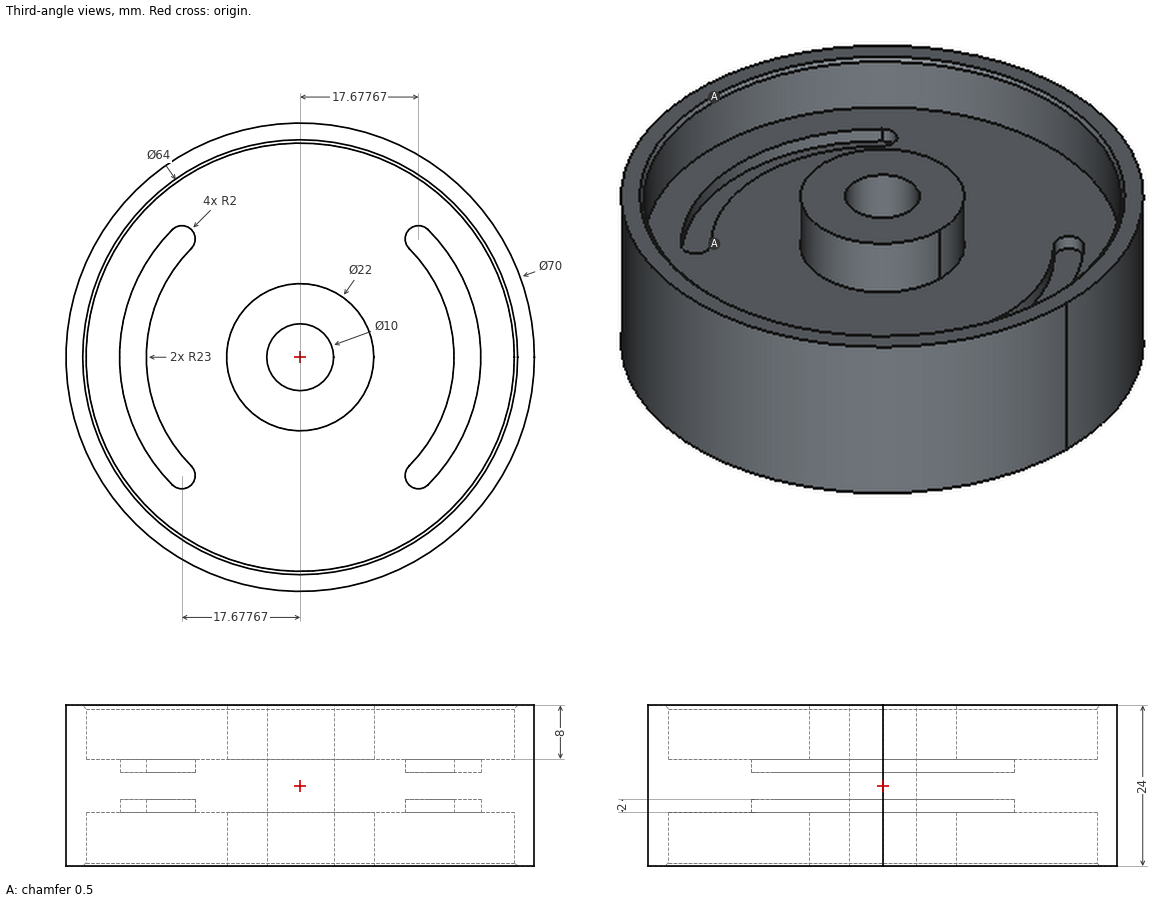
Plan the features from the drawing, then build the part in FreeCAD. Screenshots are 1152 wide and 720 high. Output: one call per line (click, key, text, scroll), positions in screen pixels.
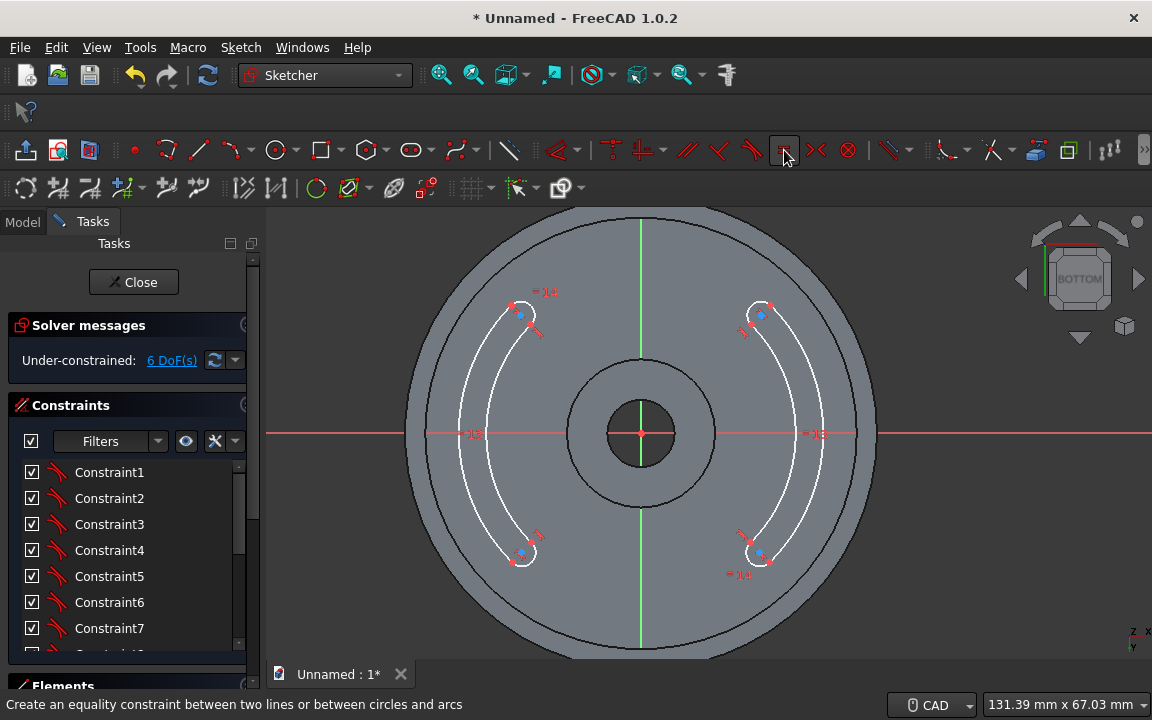
key(d)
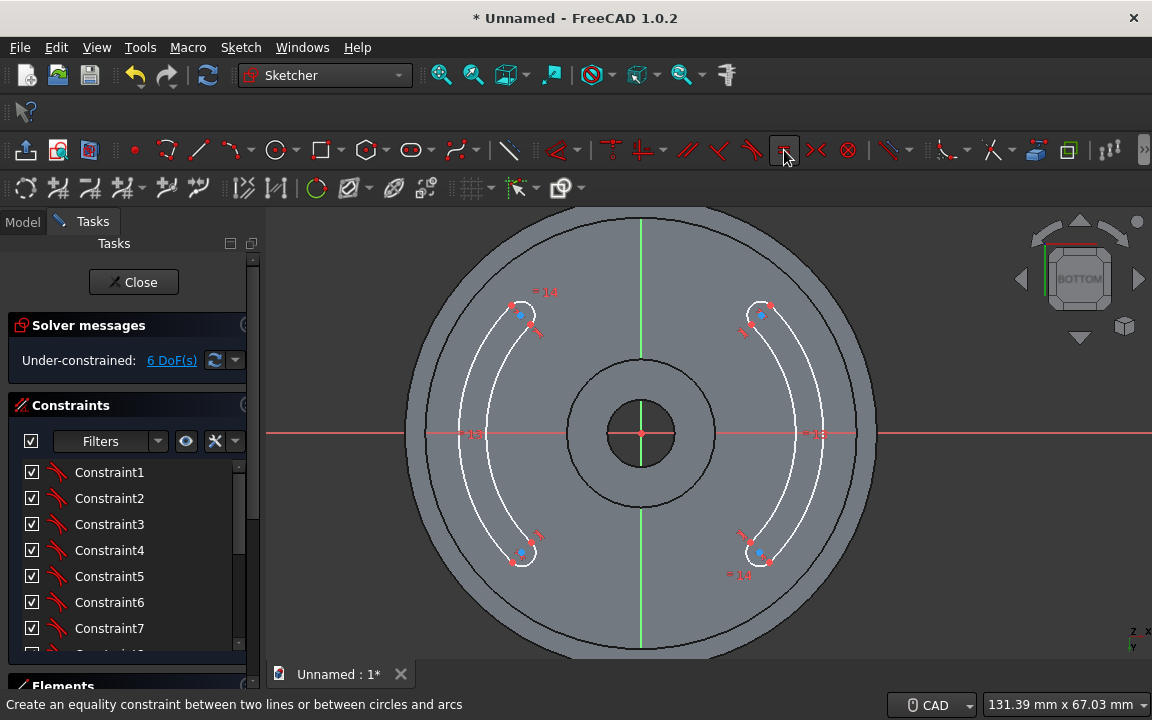
click(494, 387)
click(592, 254)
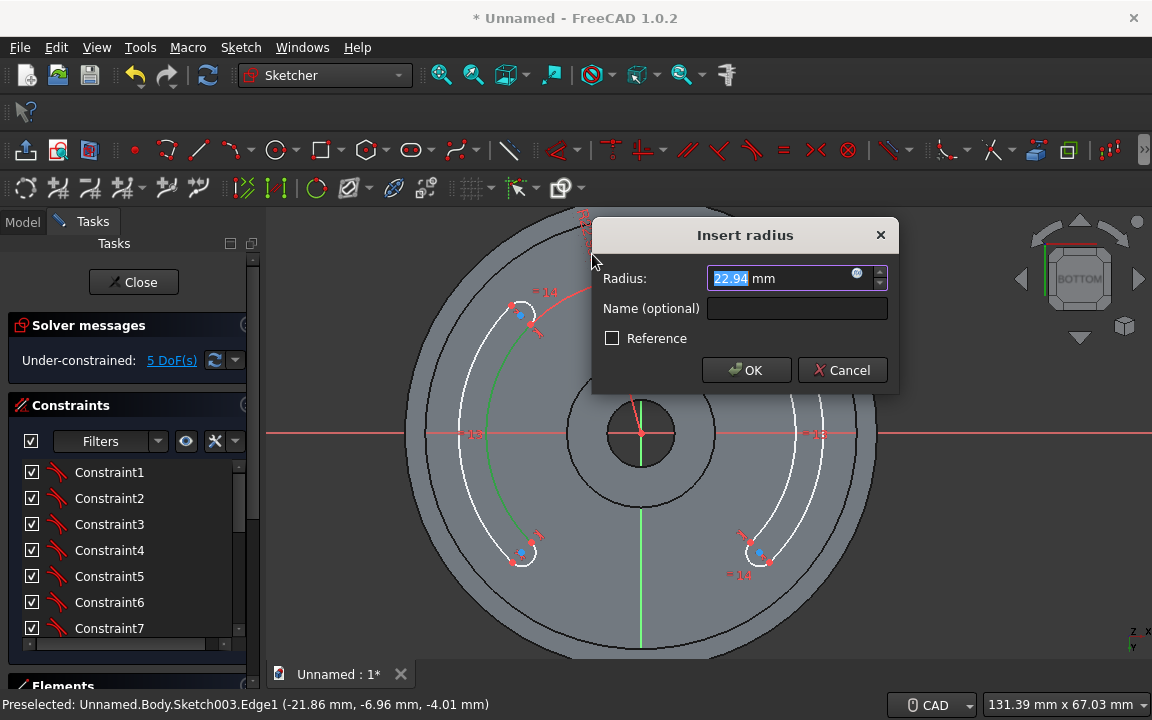
text(23)
key(Return)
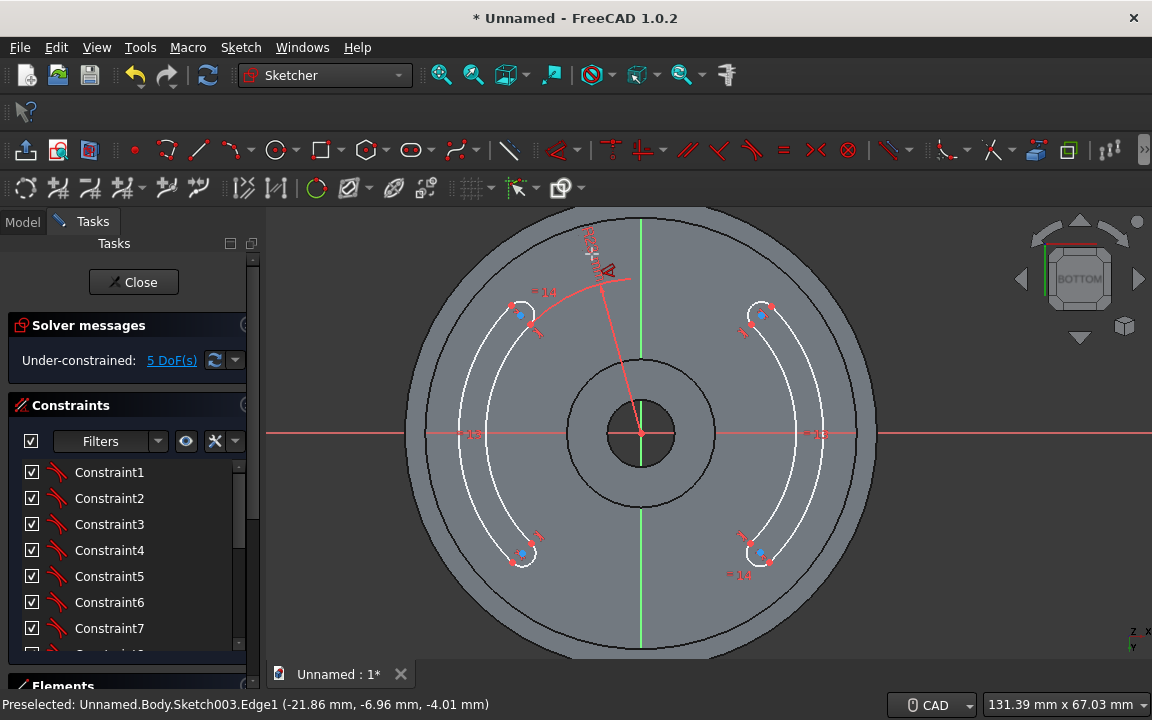
scroll(534, 313, up, 6)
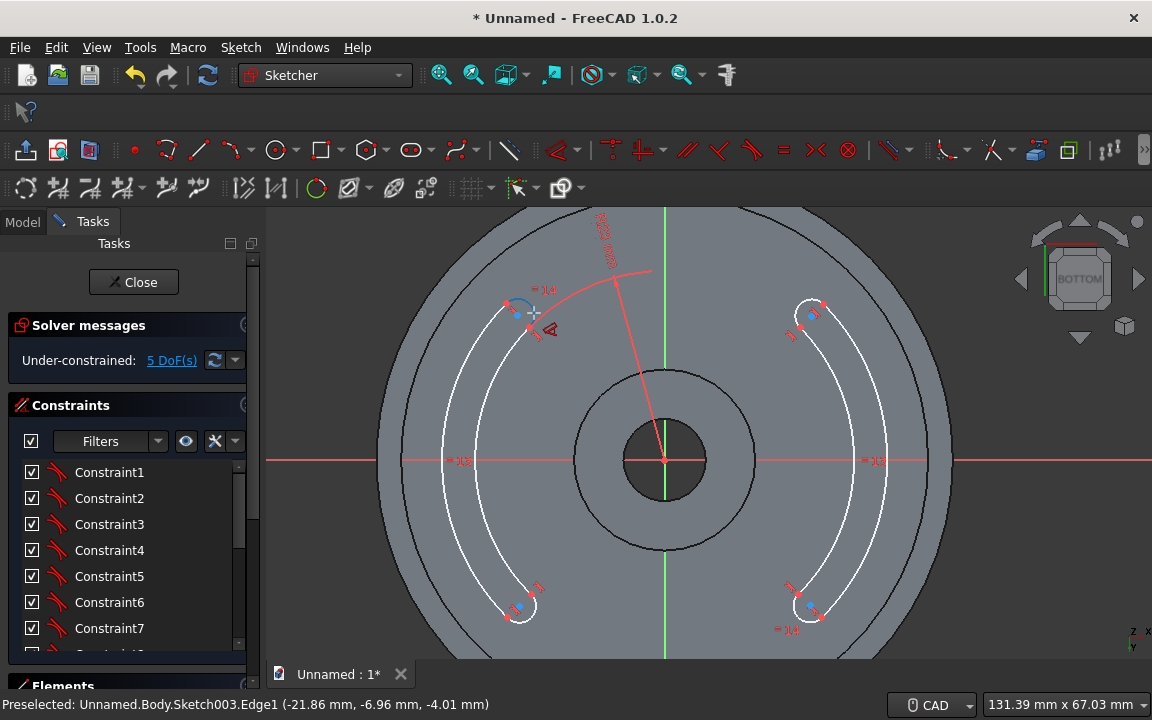
click(534, 312)
click(566, 307)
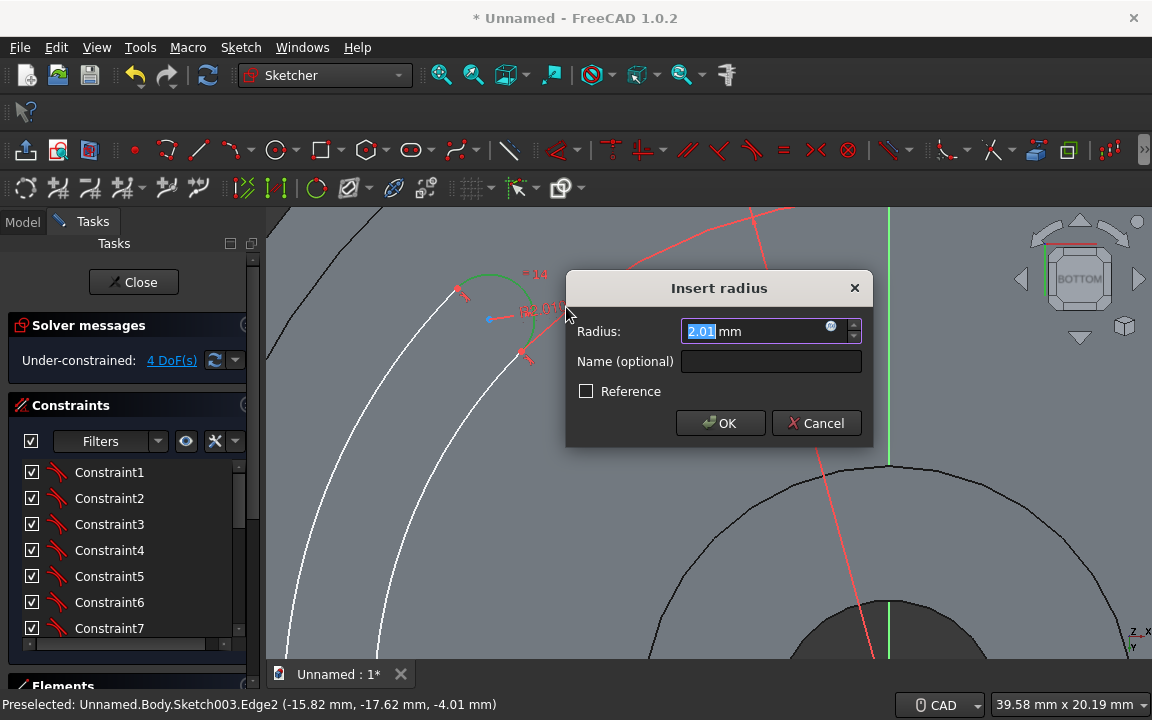
text(2)
key(Return)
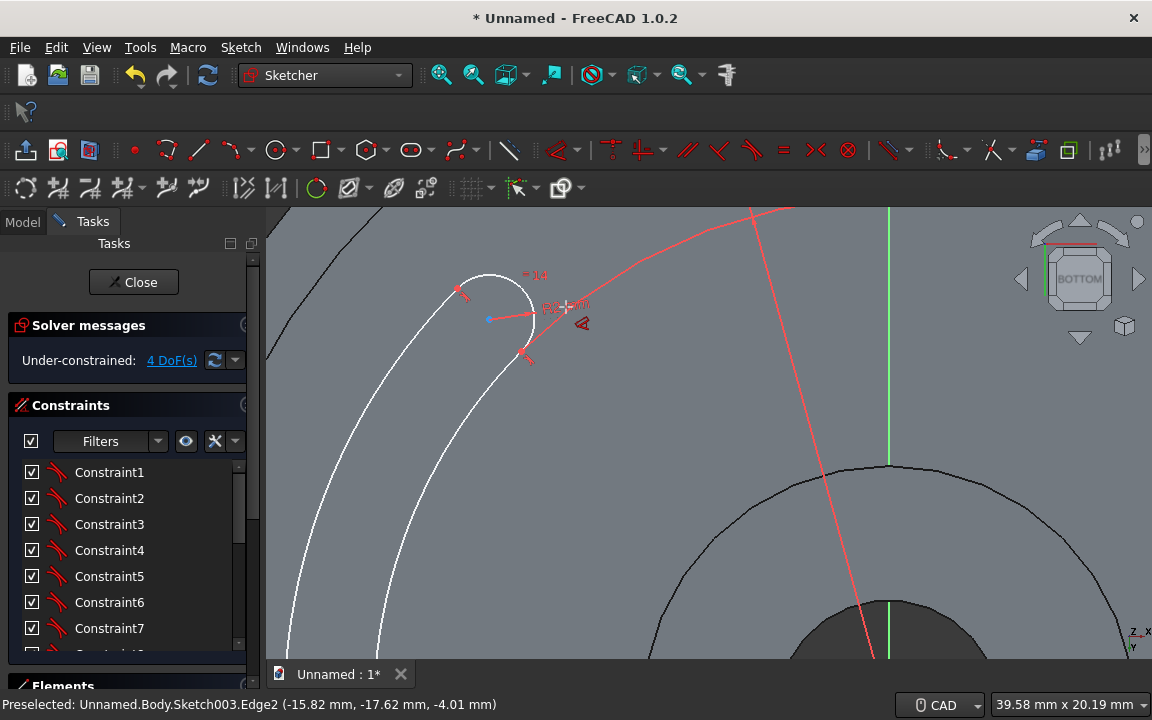
click(490, 320)
click(689, 286)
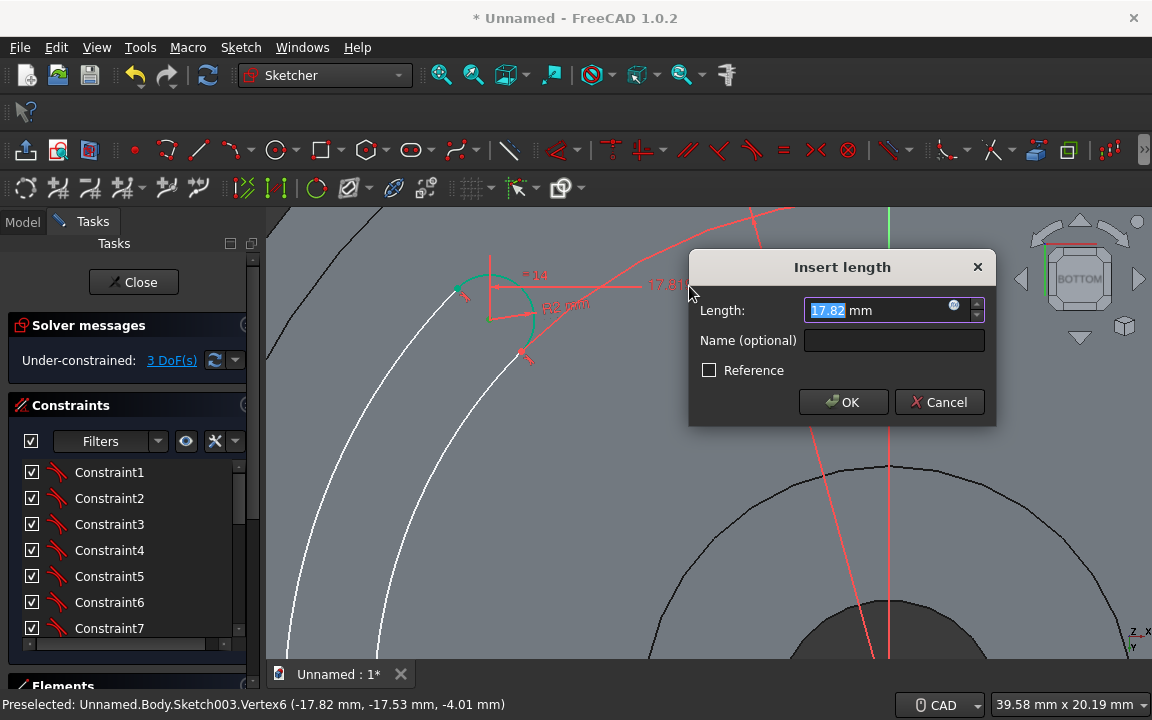
text(17.67767)
key(Return)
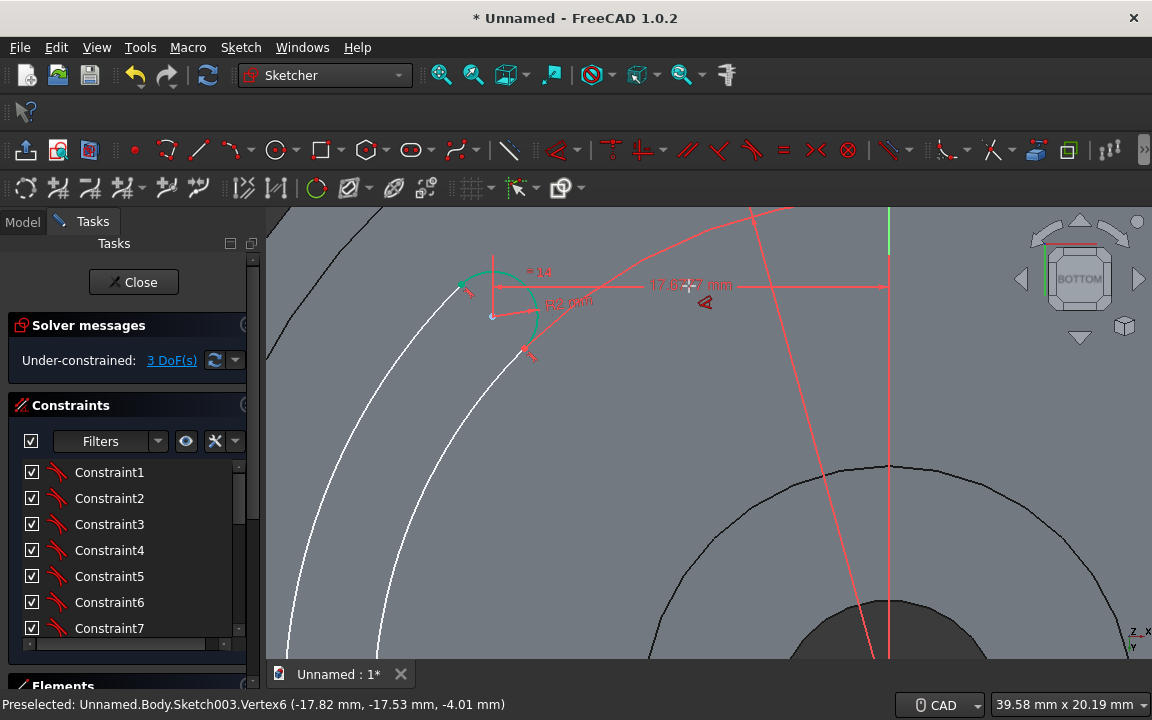
scroll(534, 313, down, 6)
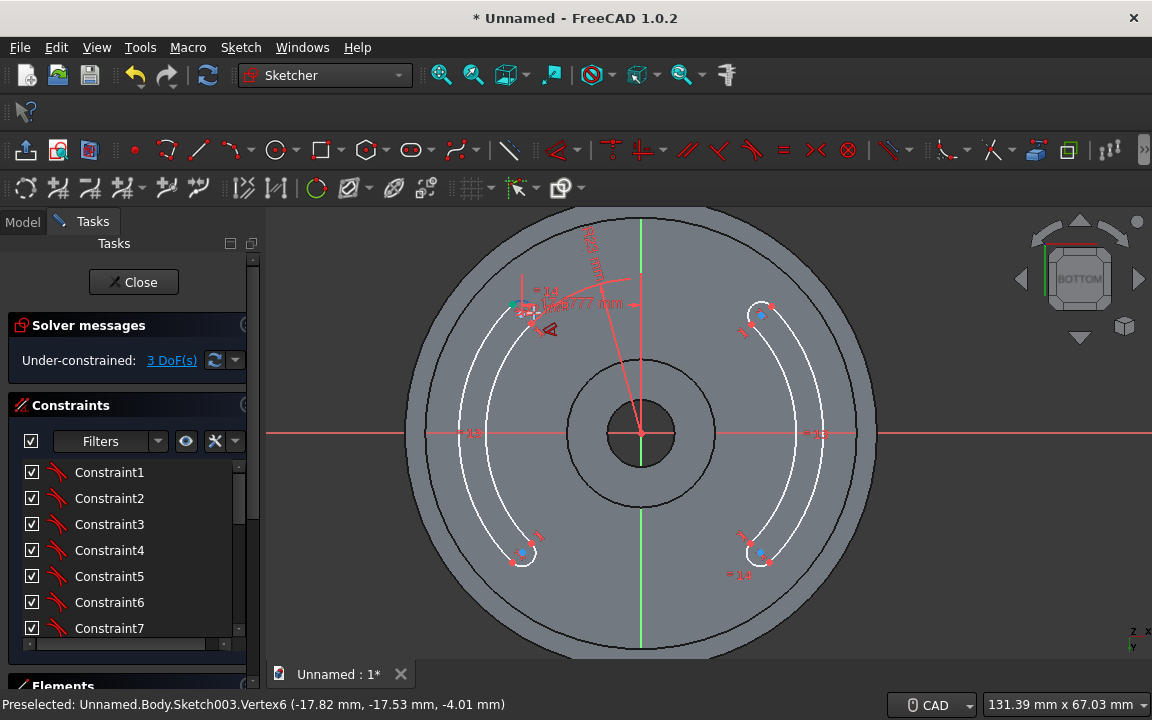
click(522, 553)
click(582, 587)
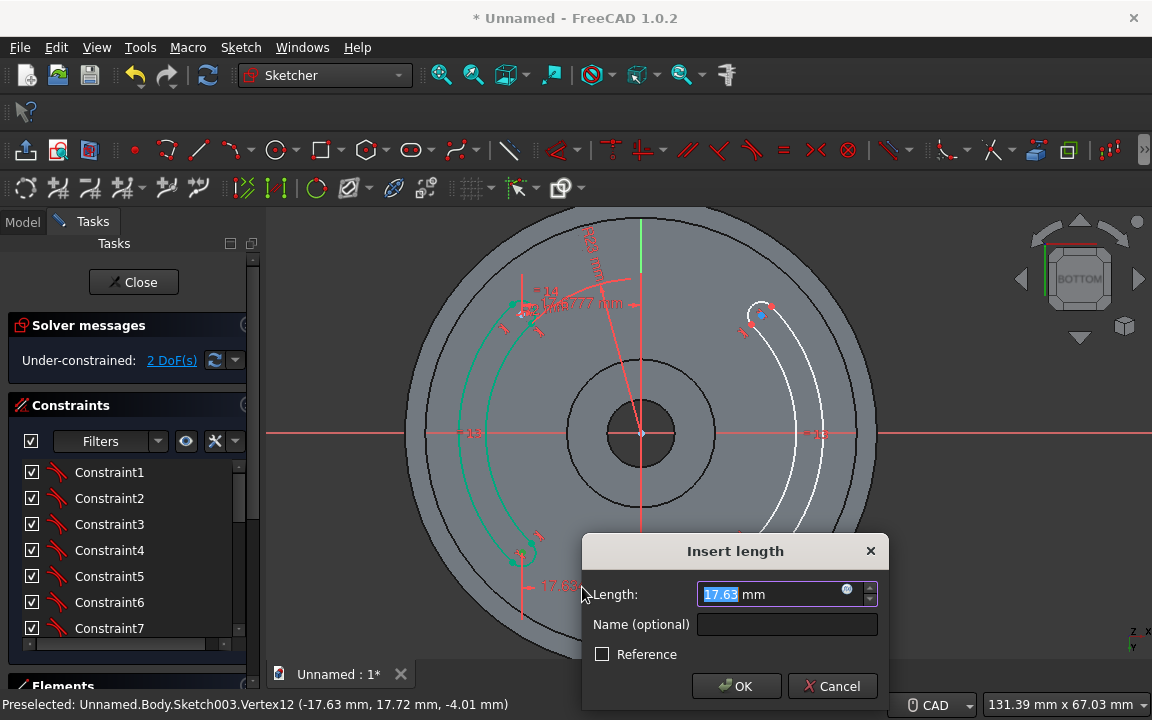
text(17.67767)
key(Return)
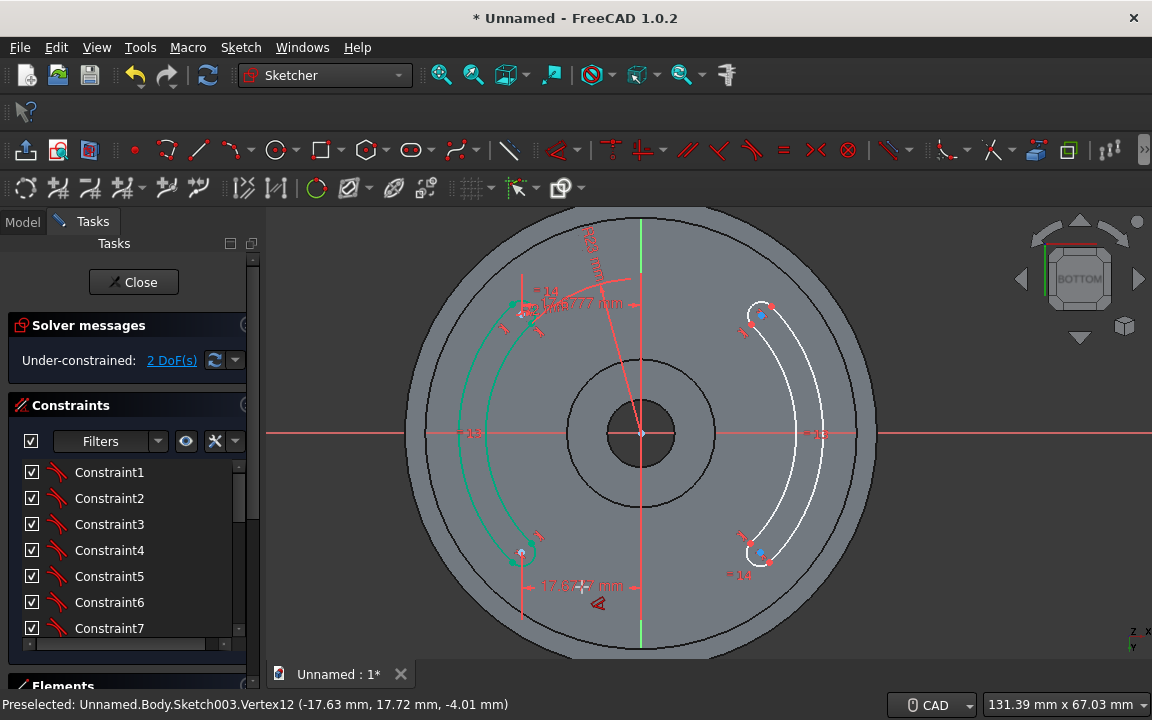
click(760, 553)
click(701, 587)